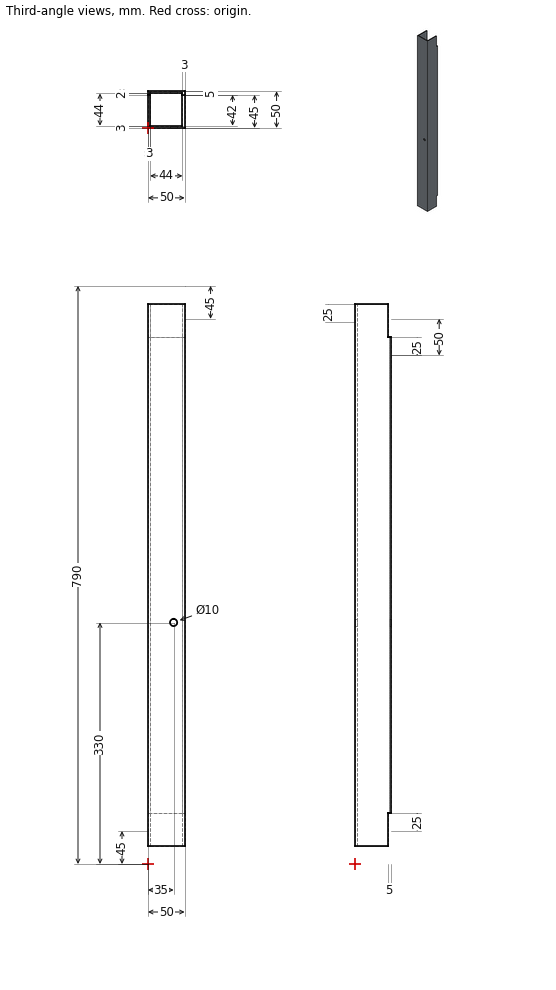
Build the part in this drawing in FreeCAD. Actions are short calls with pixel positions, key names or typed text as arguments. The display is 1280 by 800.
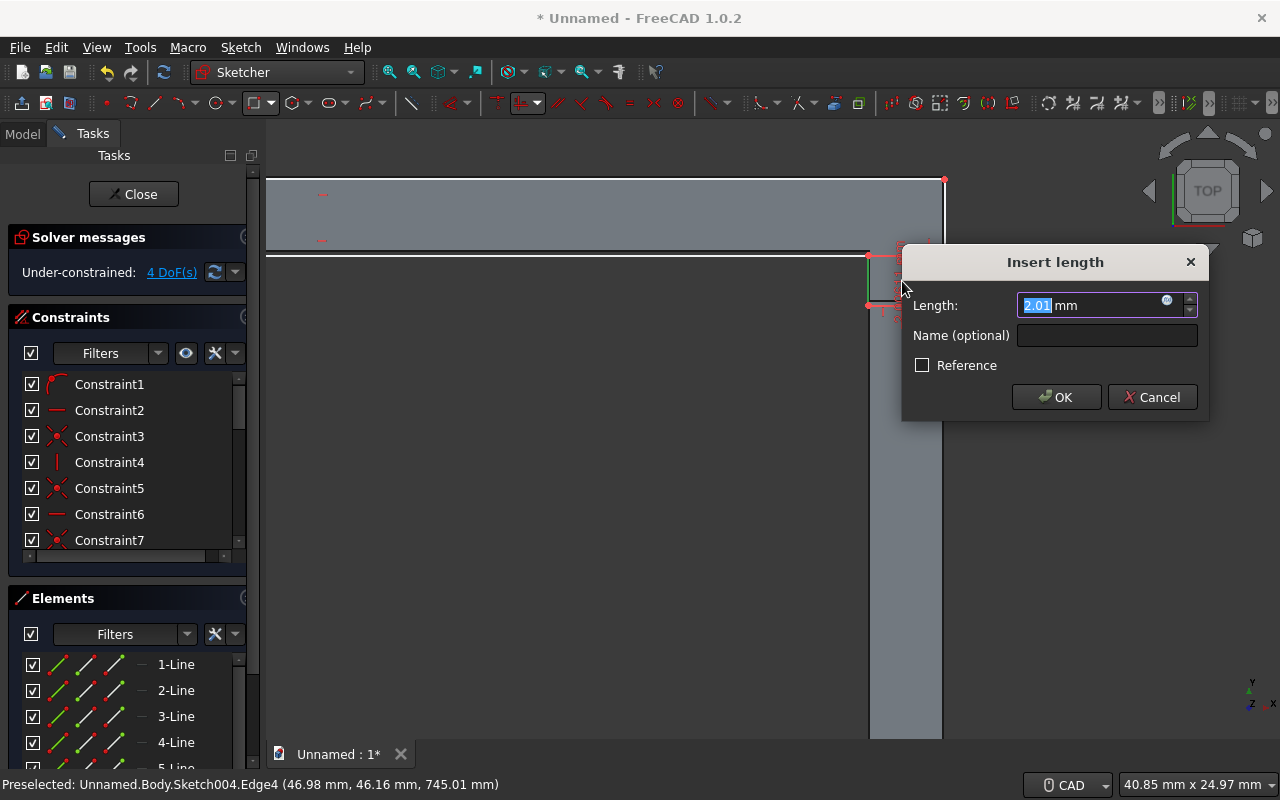
text(2)
key(Return)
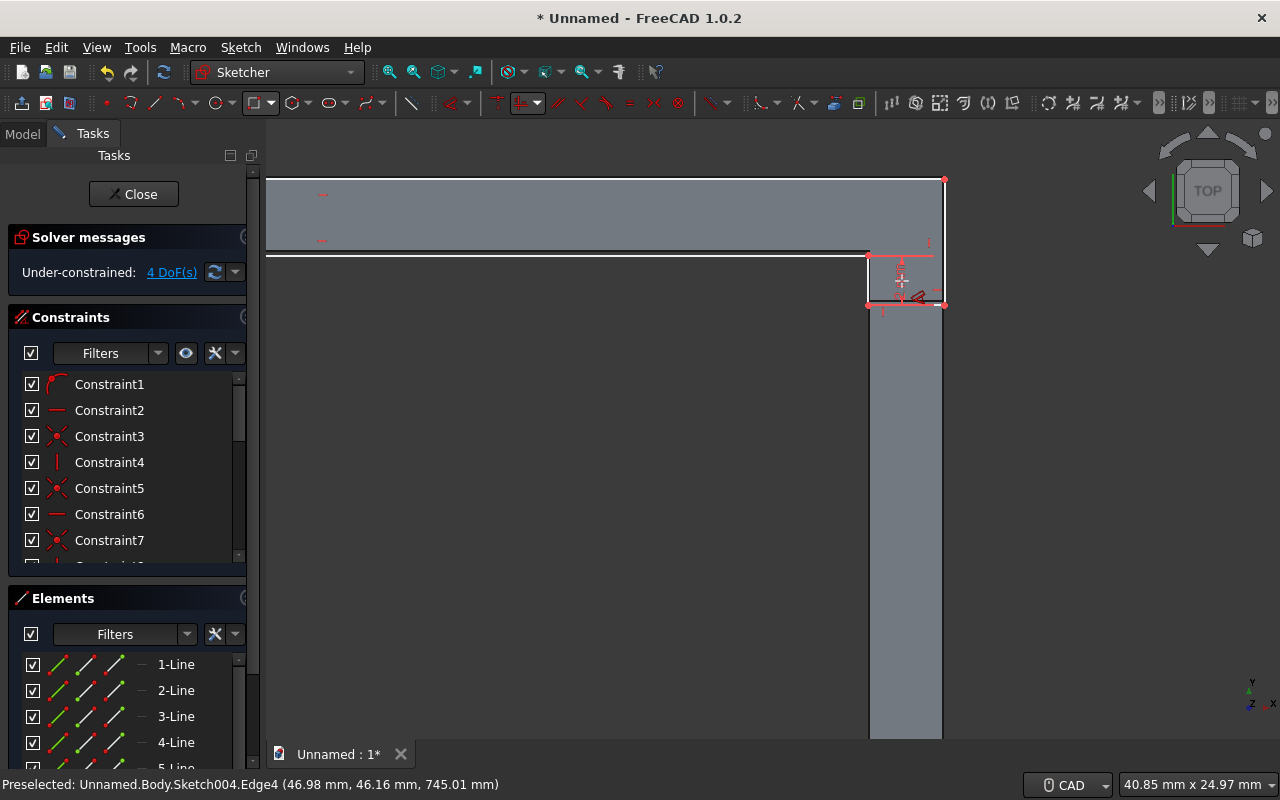
click(891, 305)
click(907, 339)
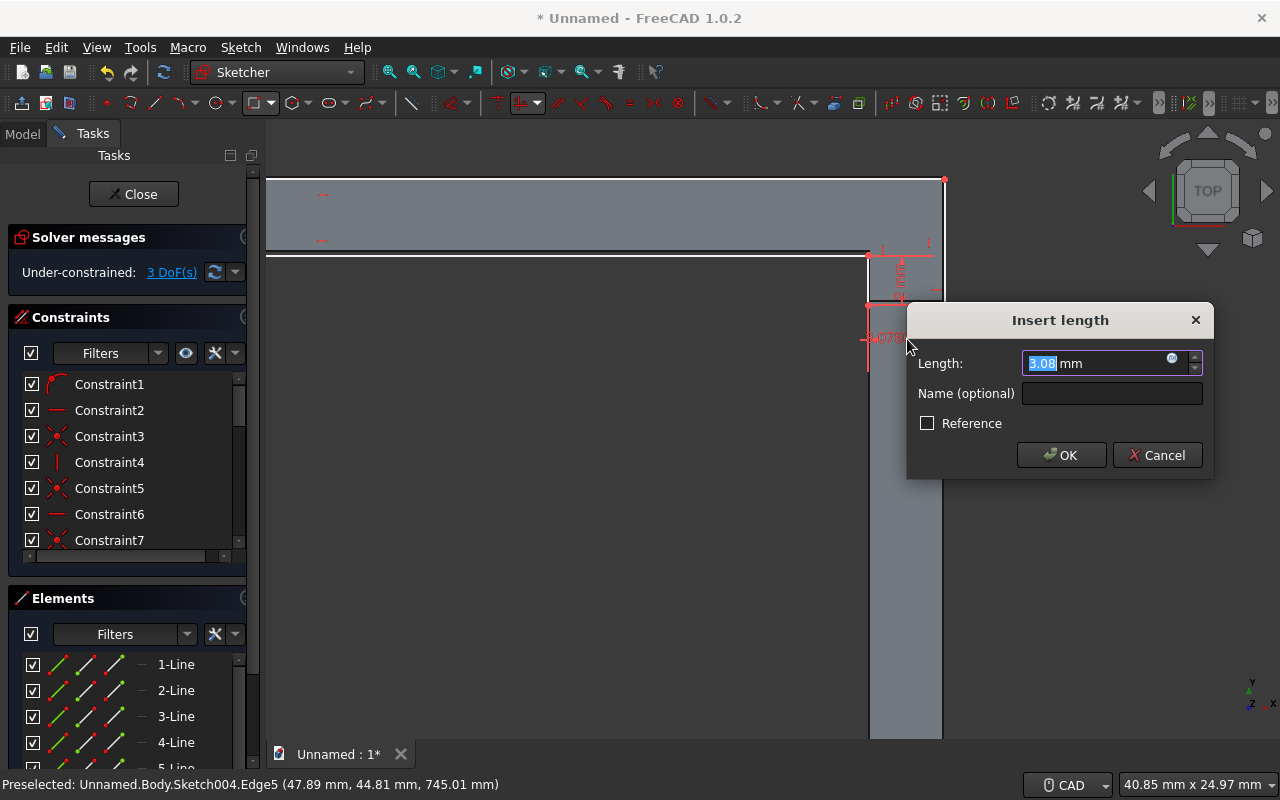
text(3)
key(Return)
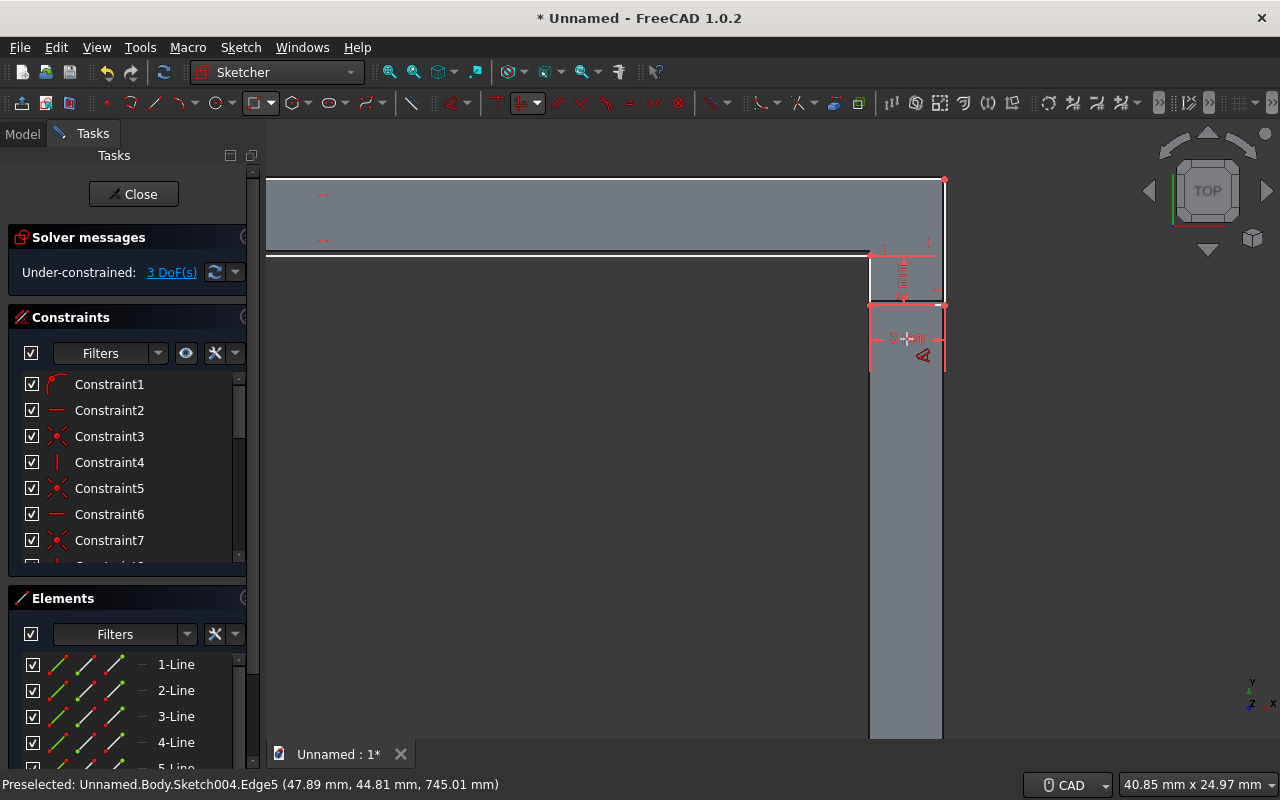
click(945, 268)
click(979, 242)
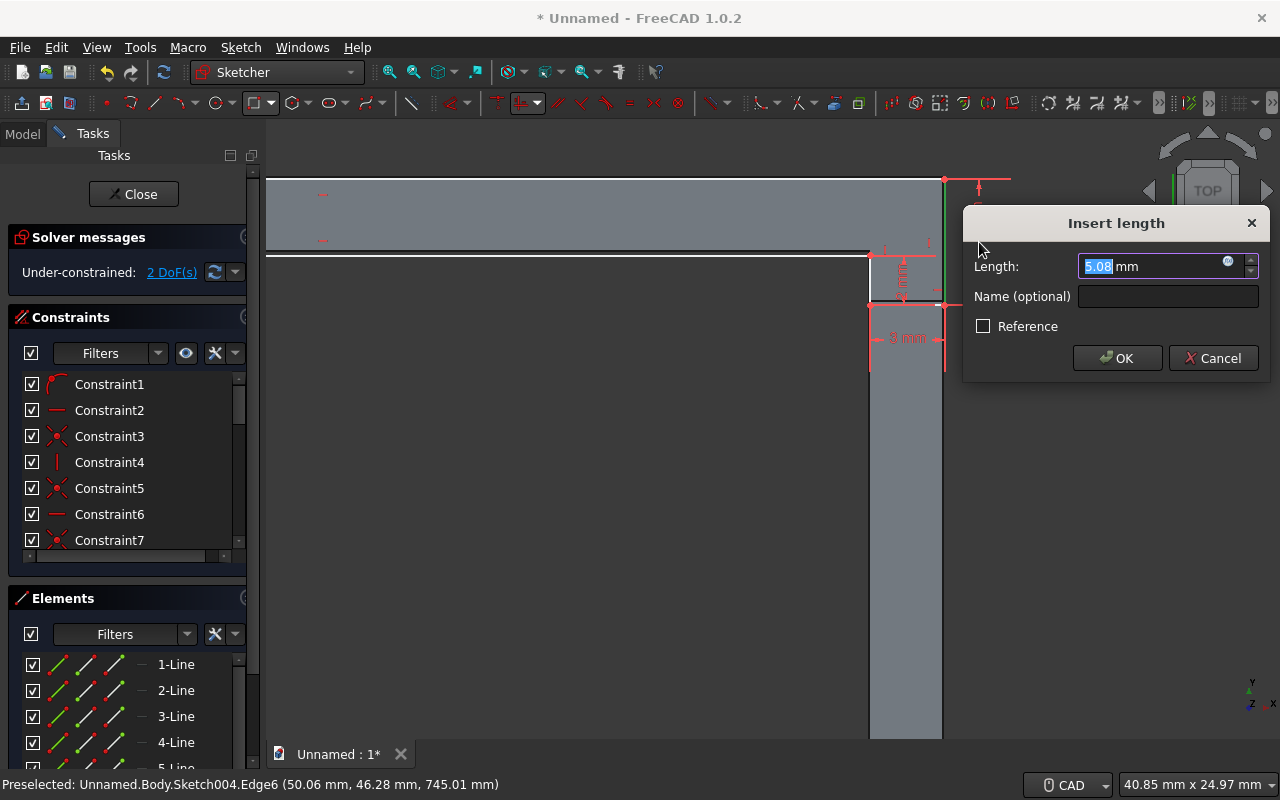
text(5)
key(Return)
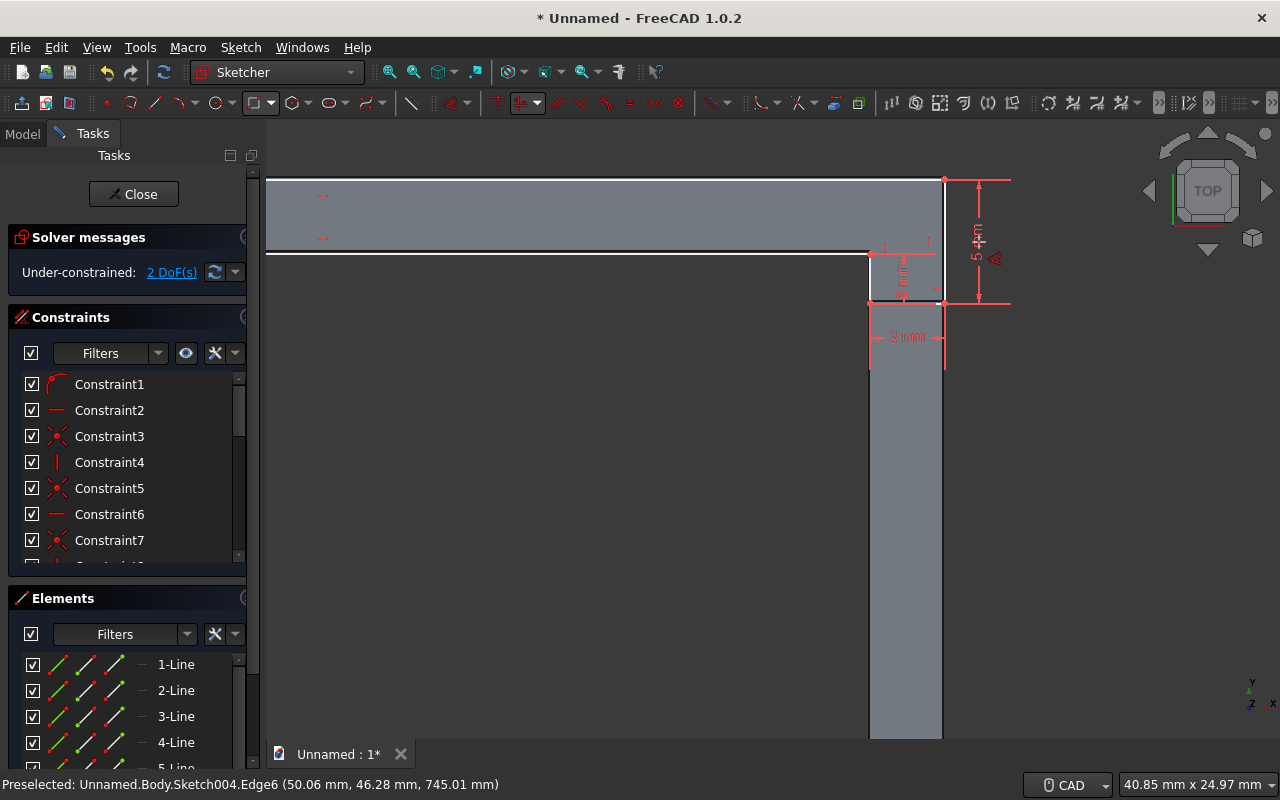
click(542, 254)
click(582, 220)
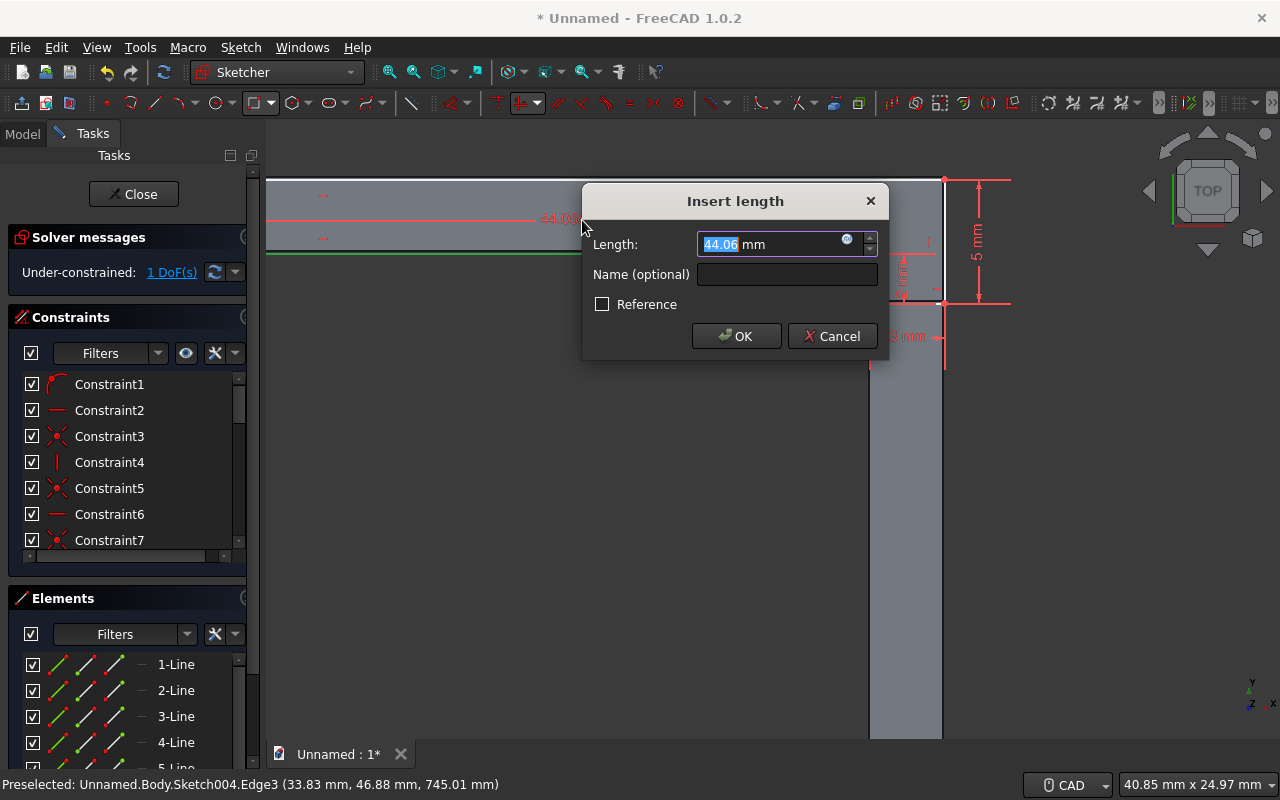
text(44)
key(Return)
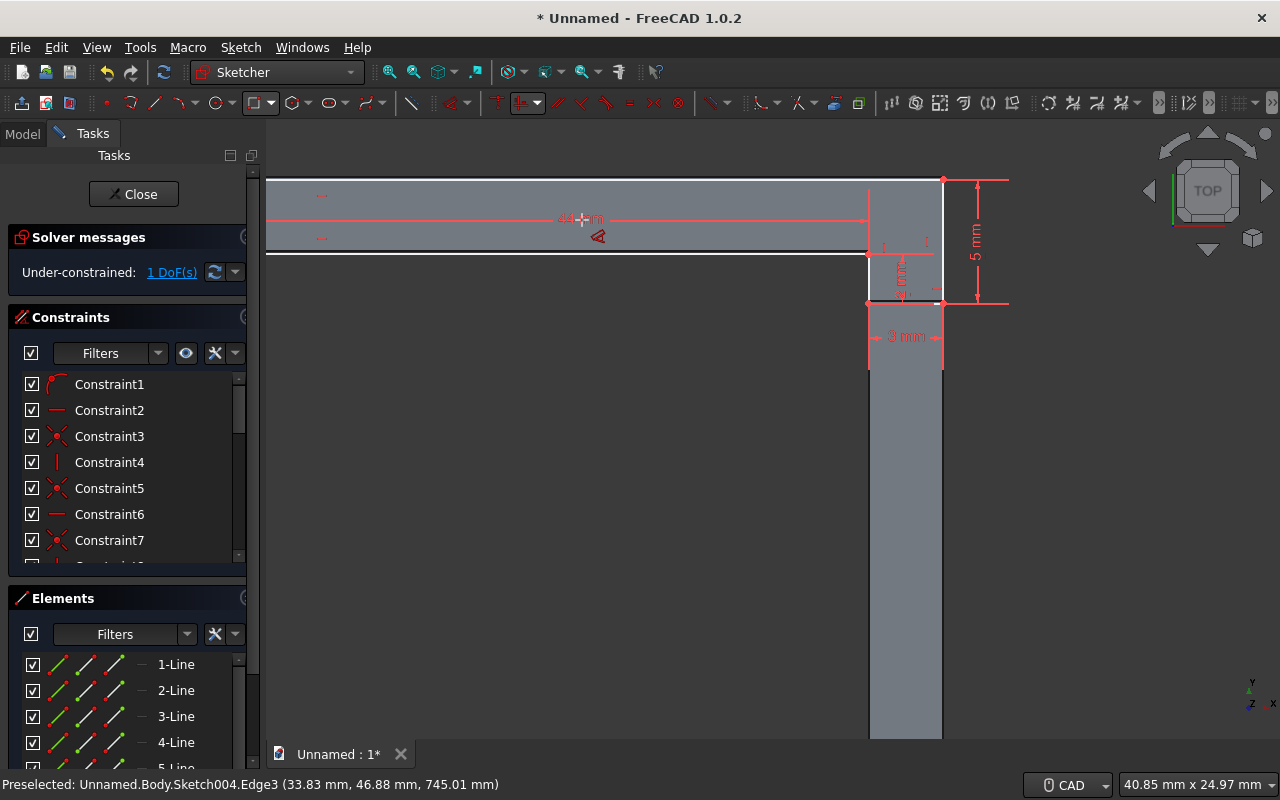
scroll(869, 270, down, 6)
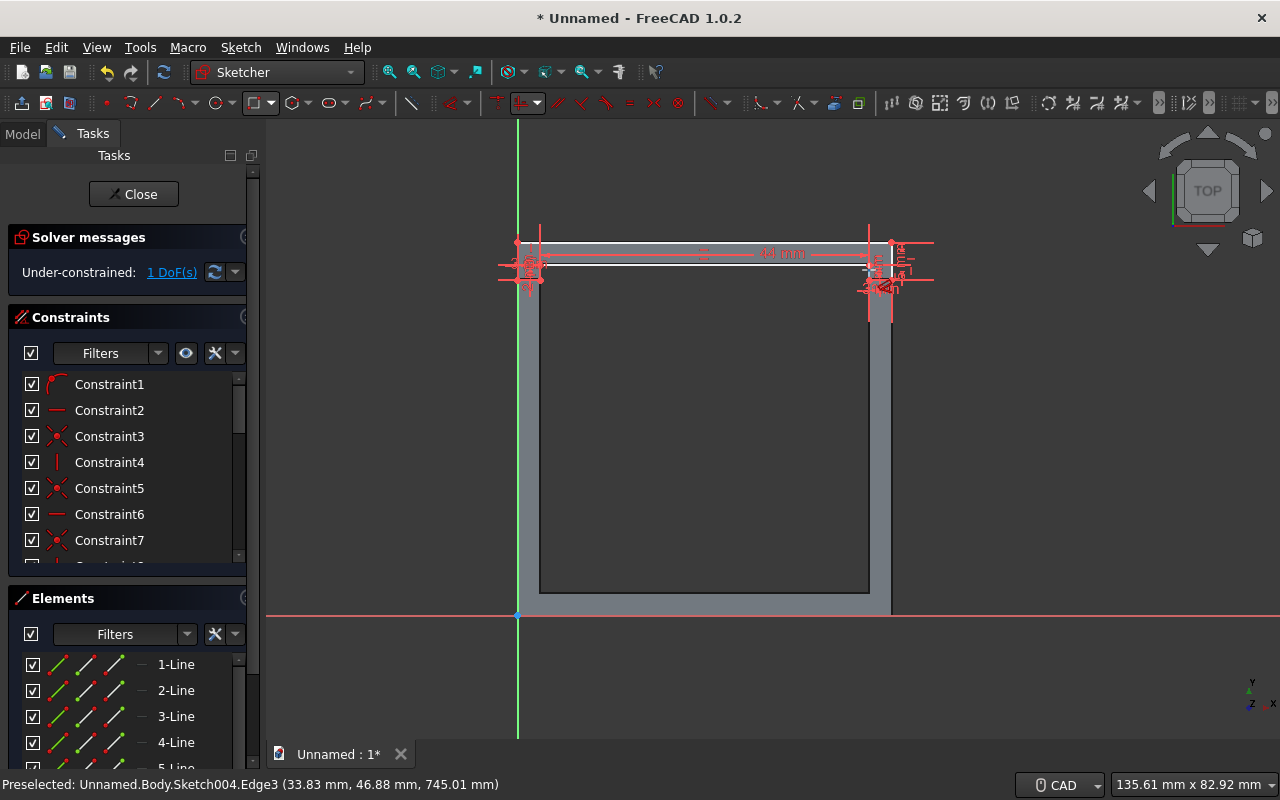
click(518, 280)
click(484, 448)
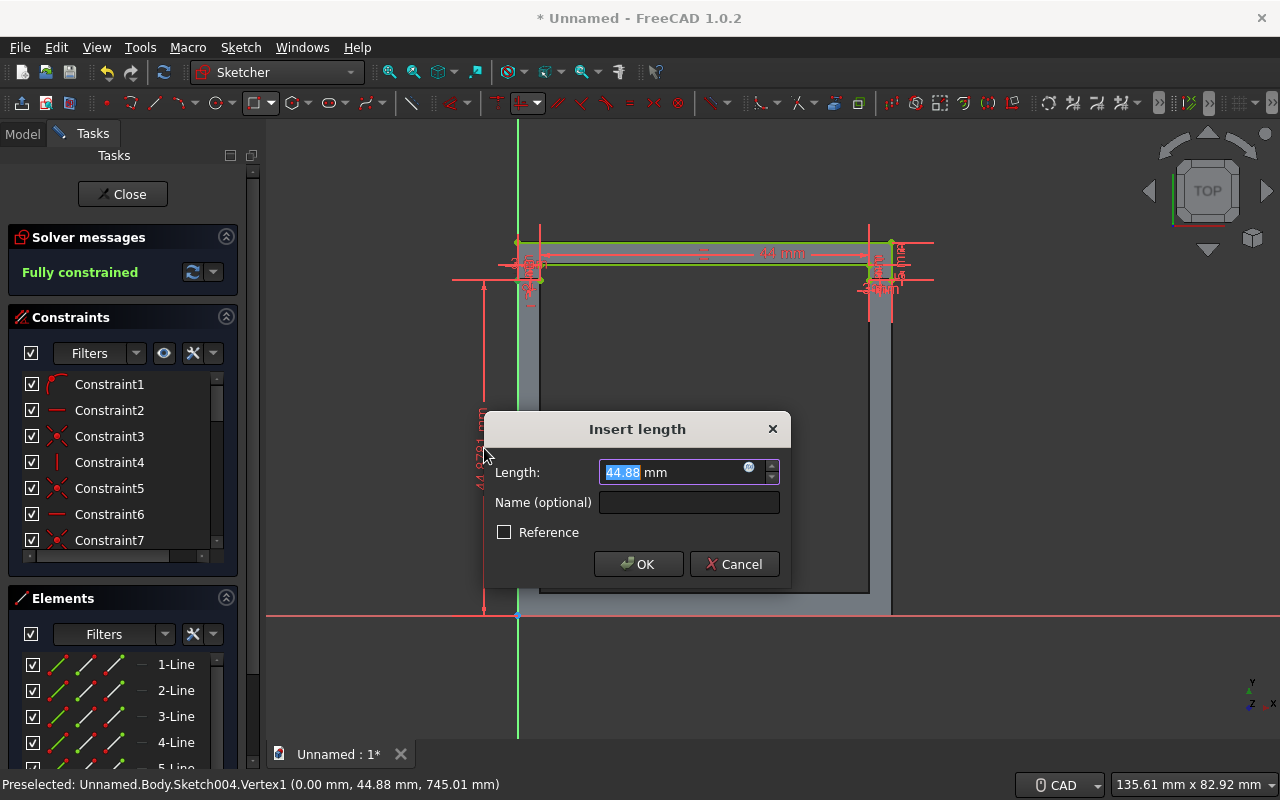
text(45)
key(Return)
key(Escape)